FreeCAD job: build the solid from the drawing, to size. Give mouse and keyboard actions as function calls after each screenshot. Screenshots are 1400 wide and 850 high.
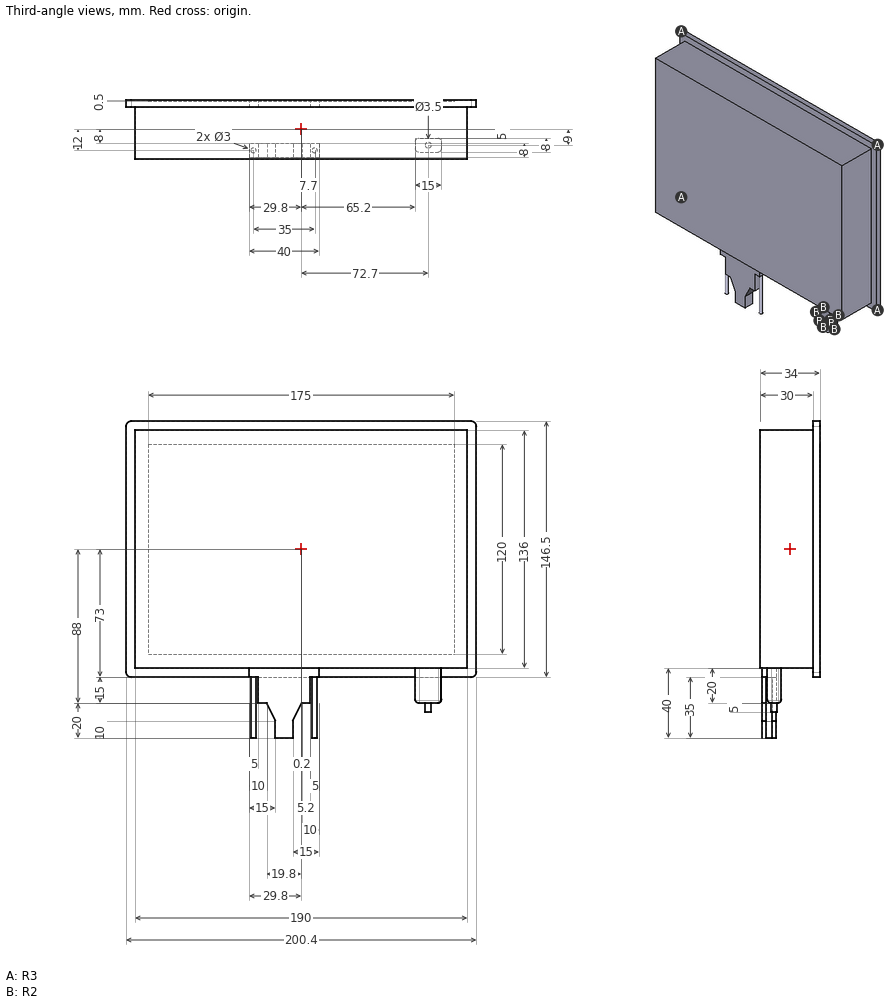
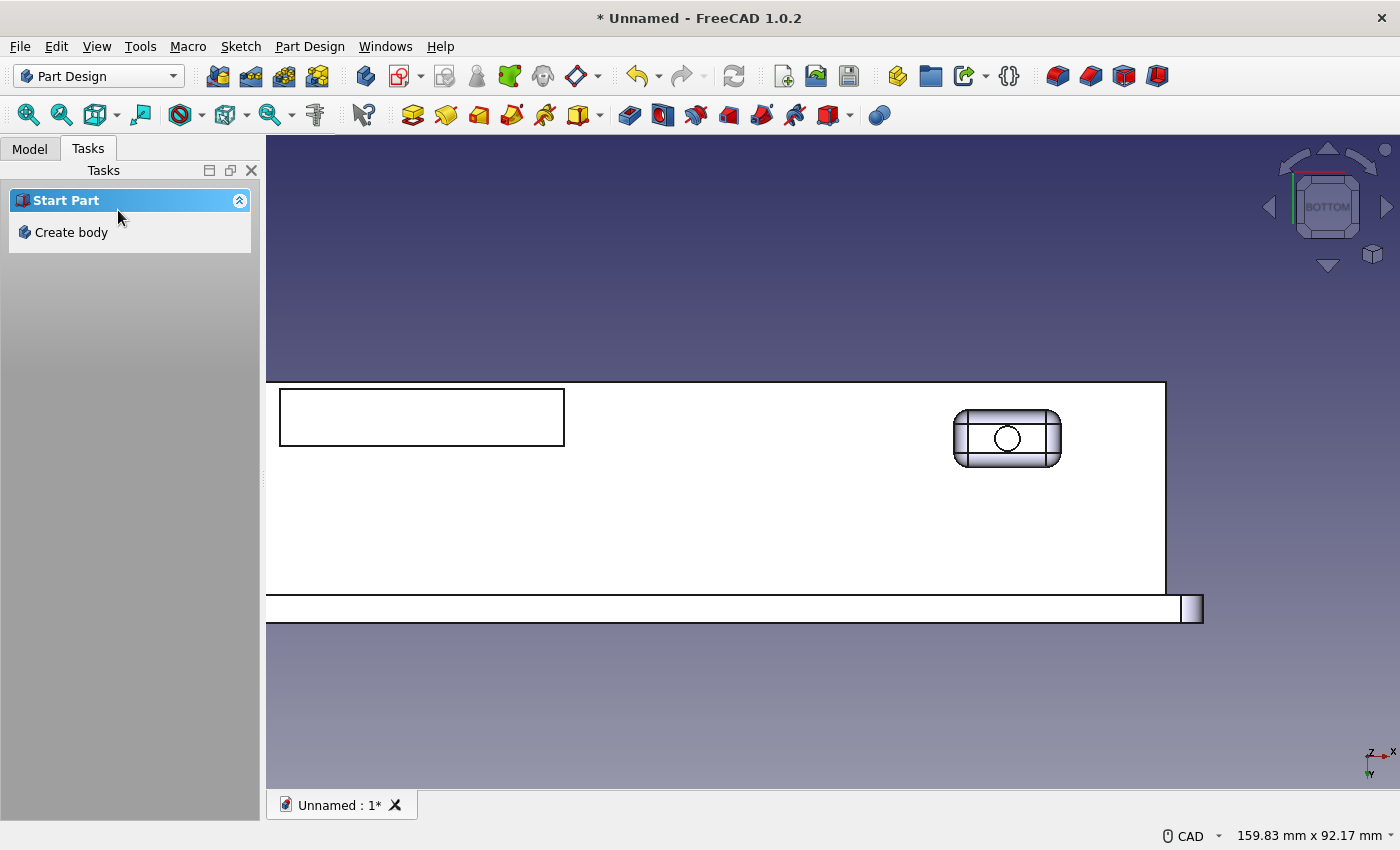
click(29, 116)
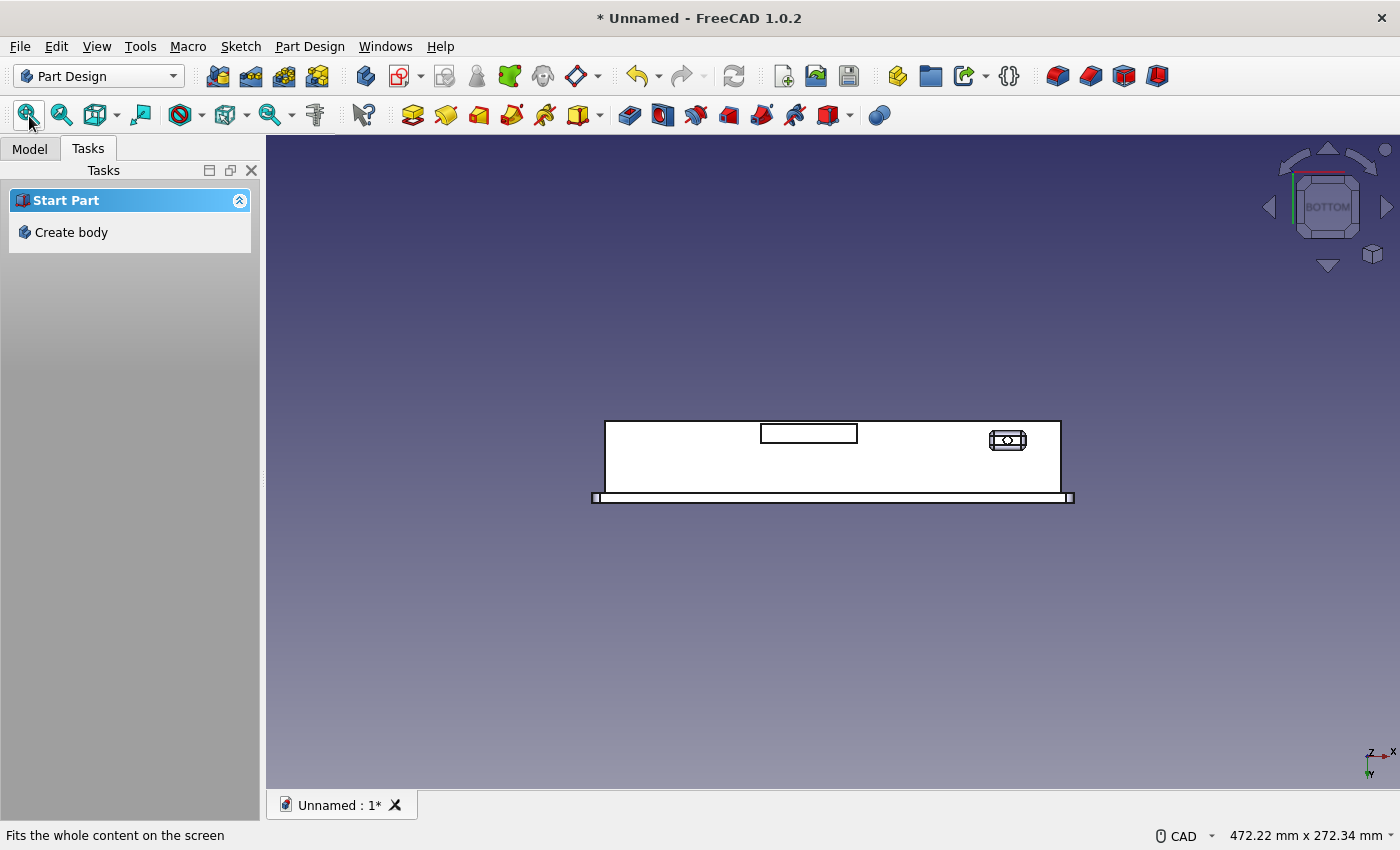
key(0)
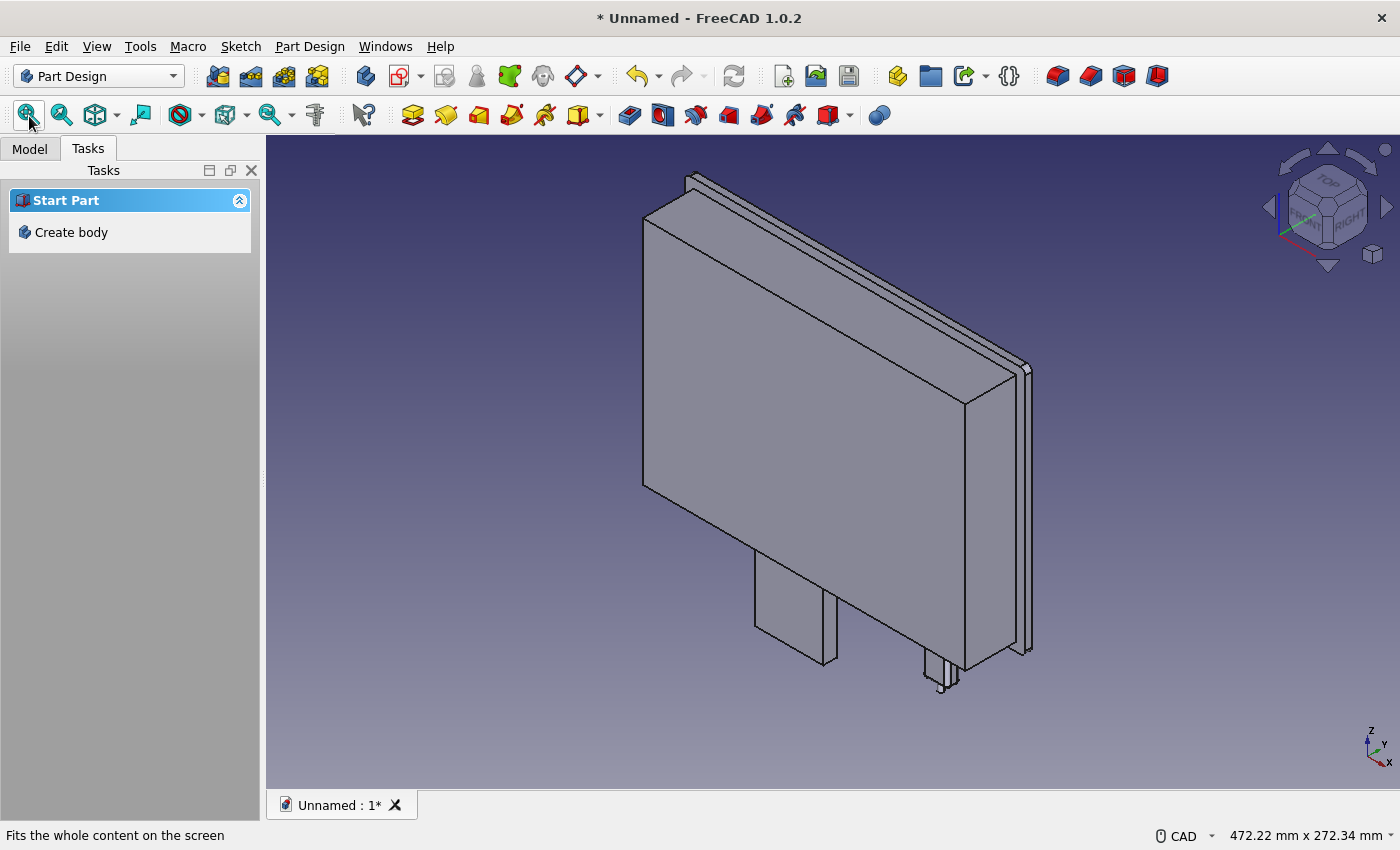
click(789, 606)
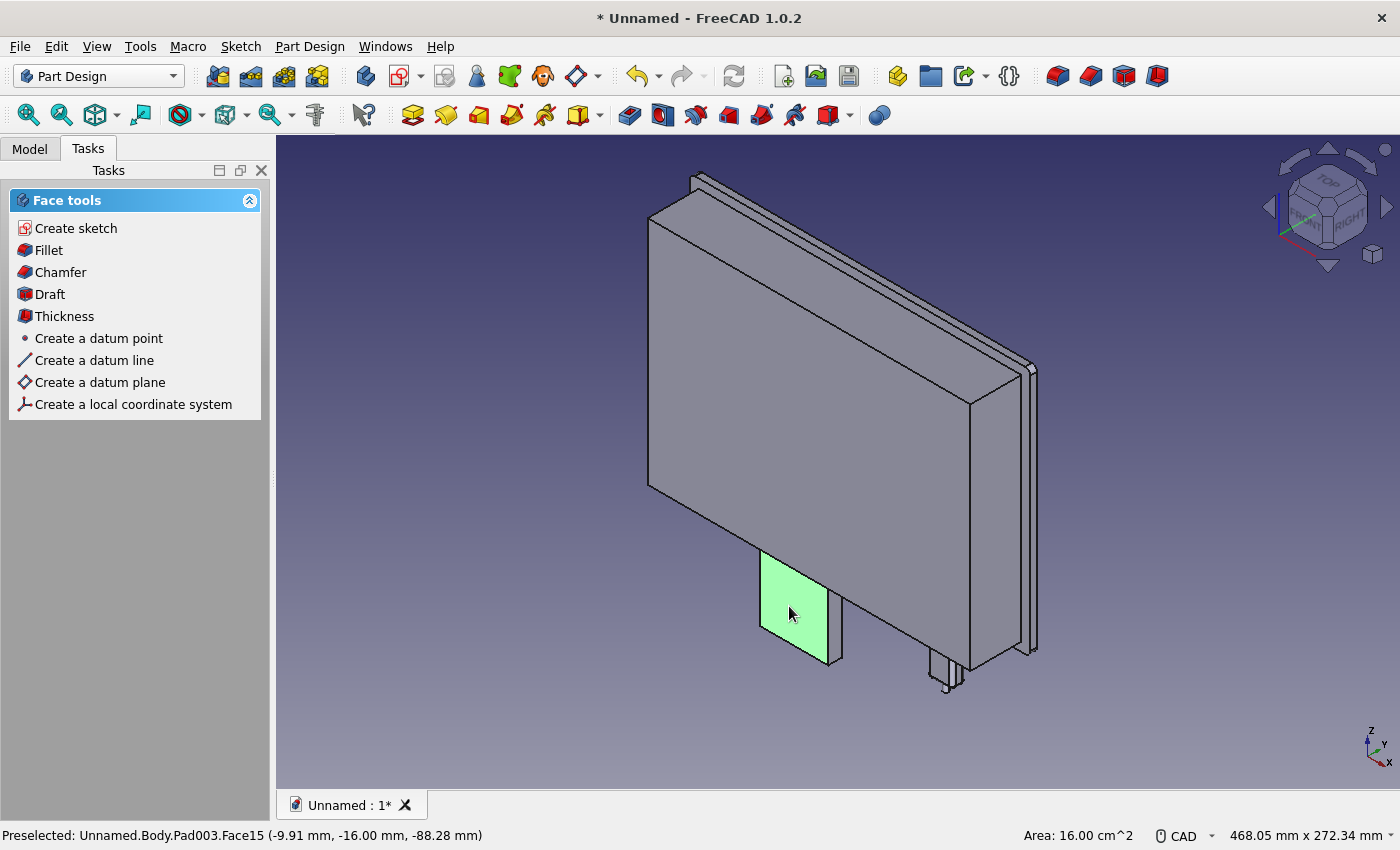
click(398, 76)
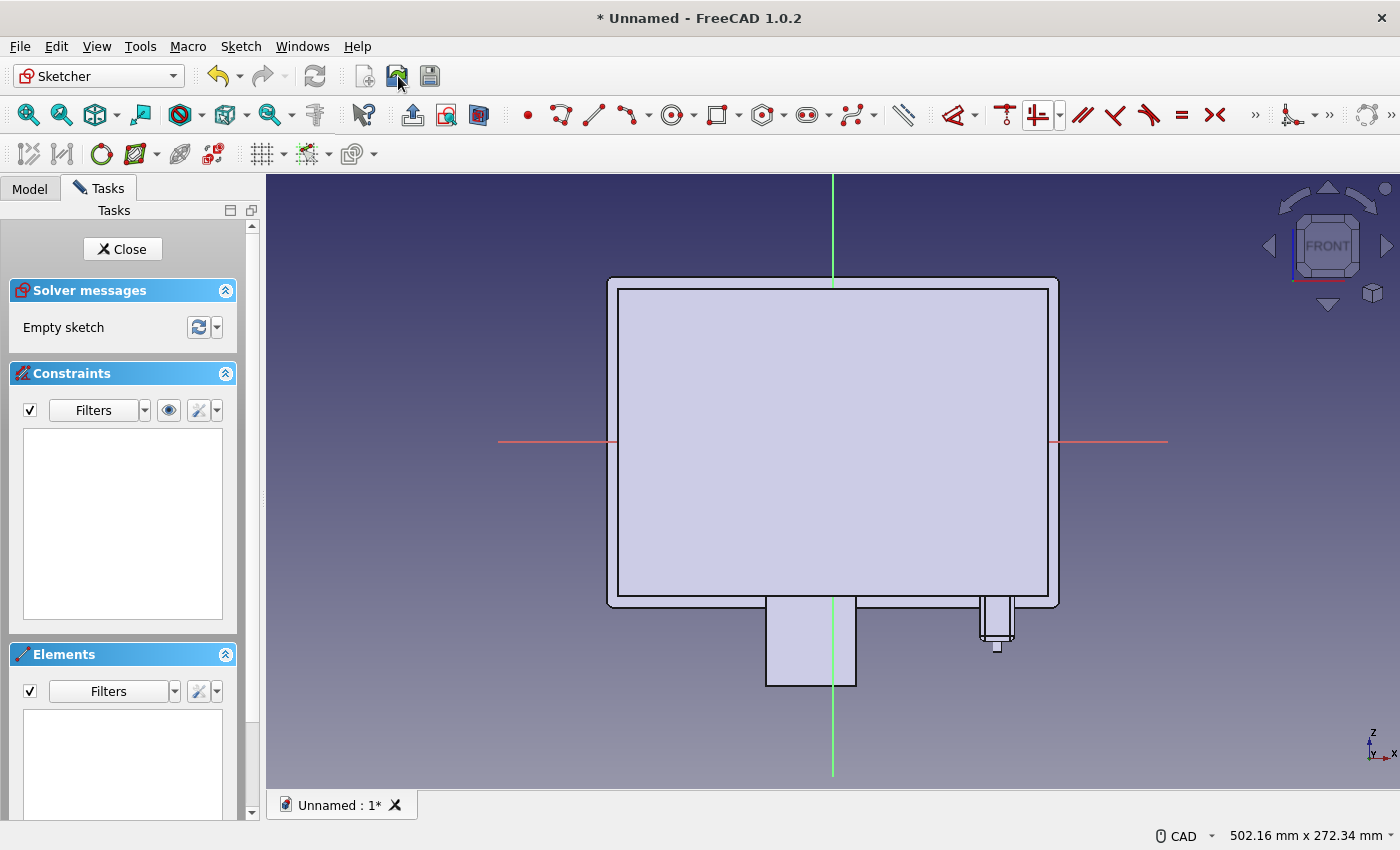
scroll(818, 692, up, 10)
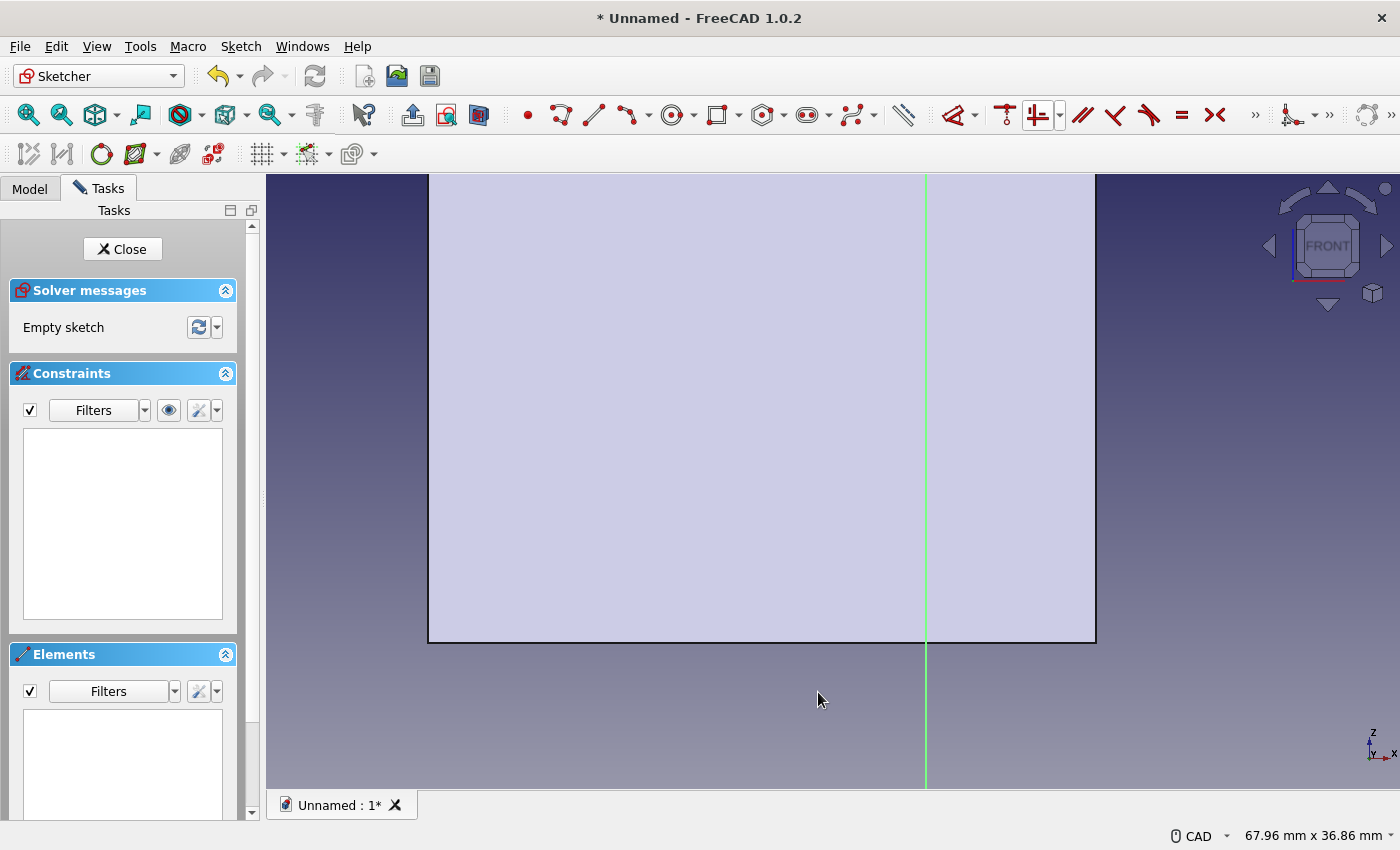
click(561, 116)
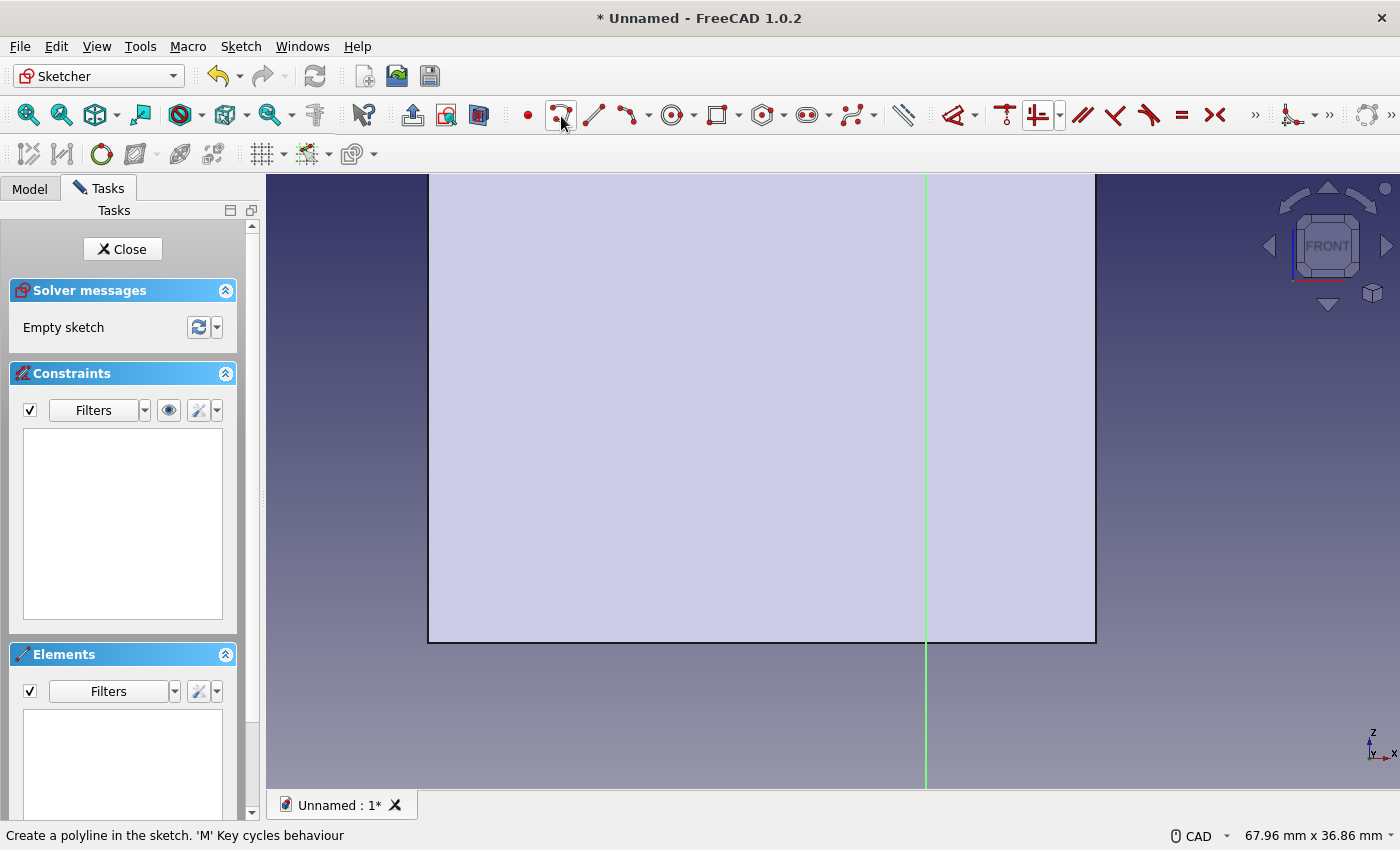
click(595, 310)
click(428, 310)
click(428, 643)
click(679, 643)
click(679, 477)
click(595, 311)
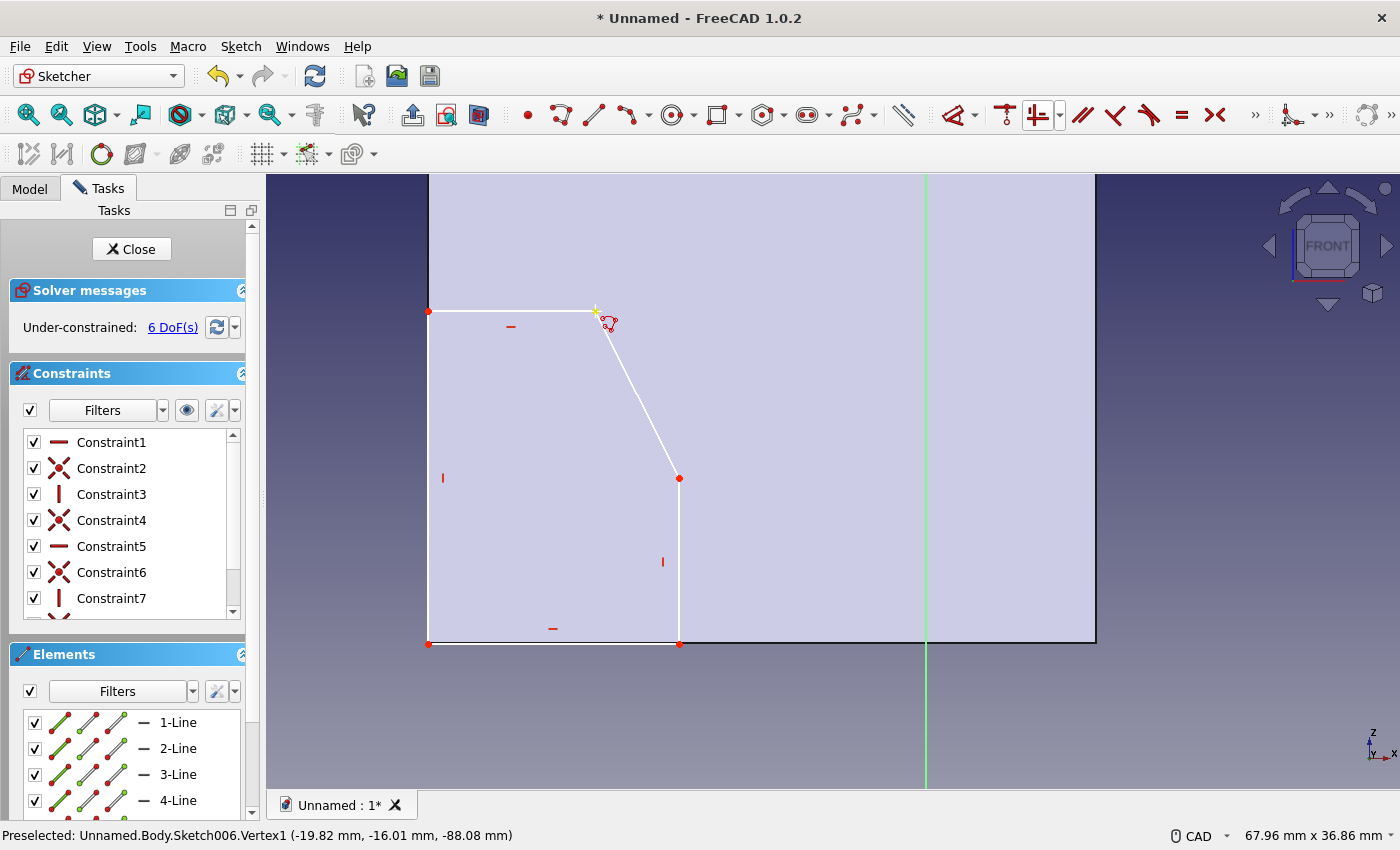
scroll(929, 310, up, 8)